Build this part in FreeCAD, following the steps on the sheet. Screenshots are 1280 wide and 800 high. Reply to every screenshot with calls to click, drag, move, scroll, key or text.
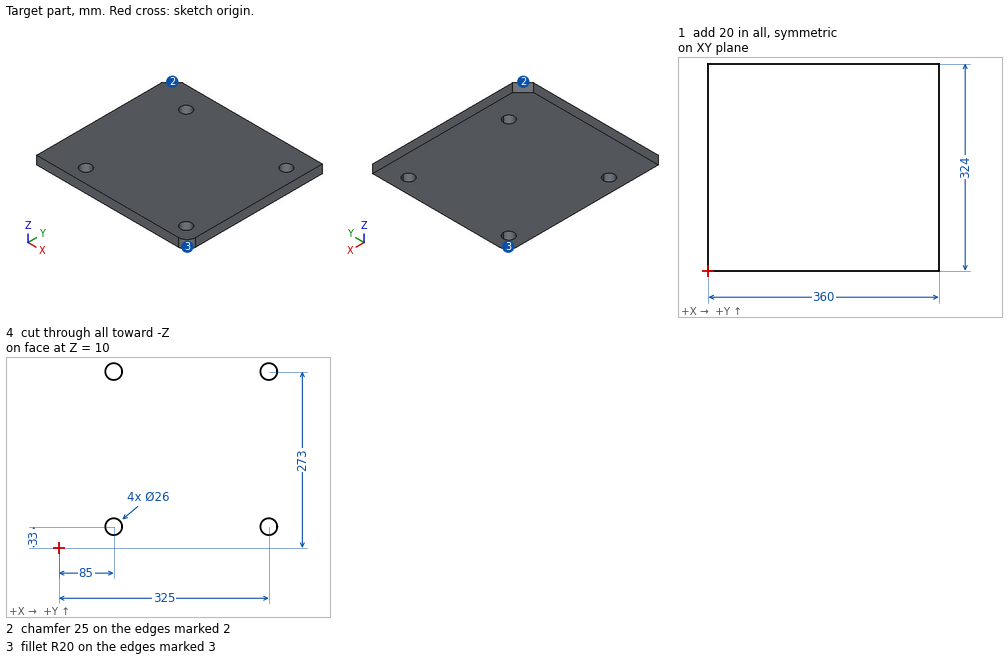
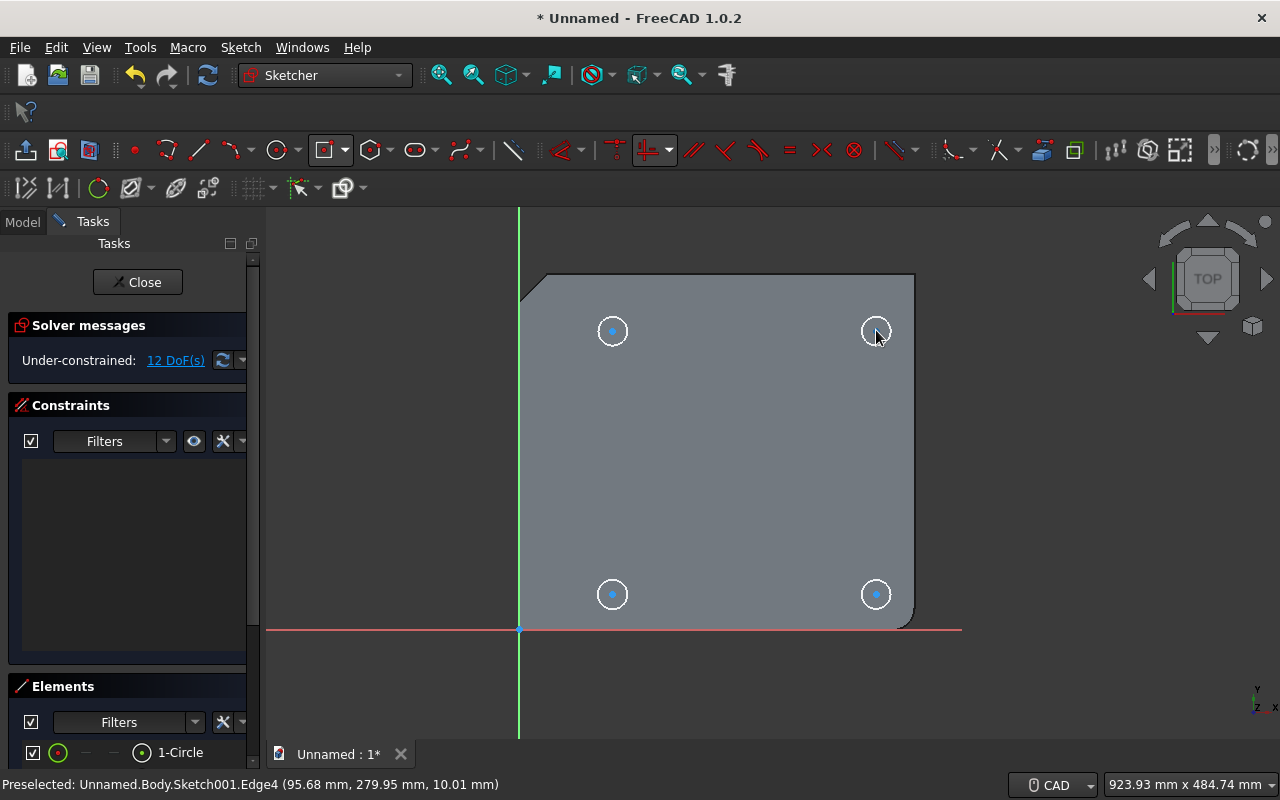
click(623, 584)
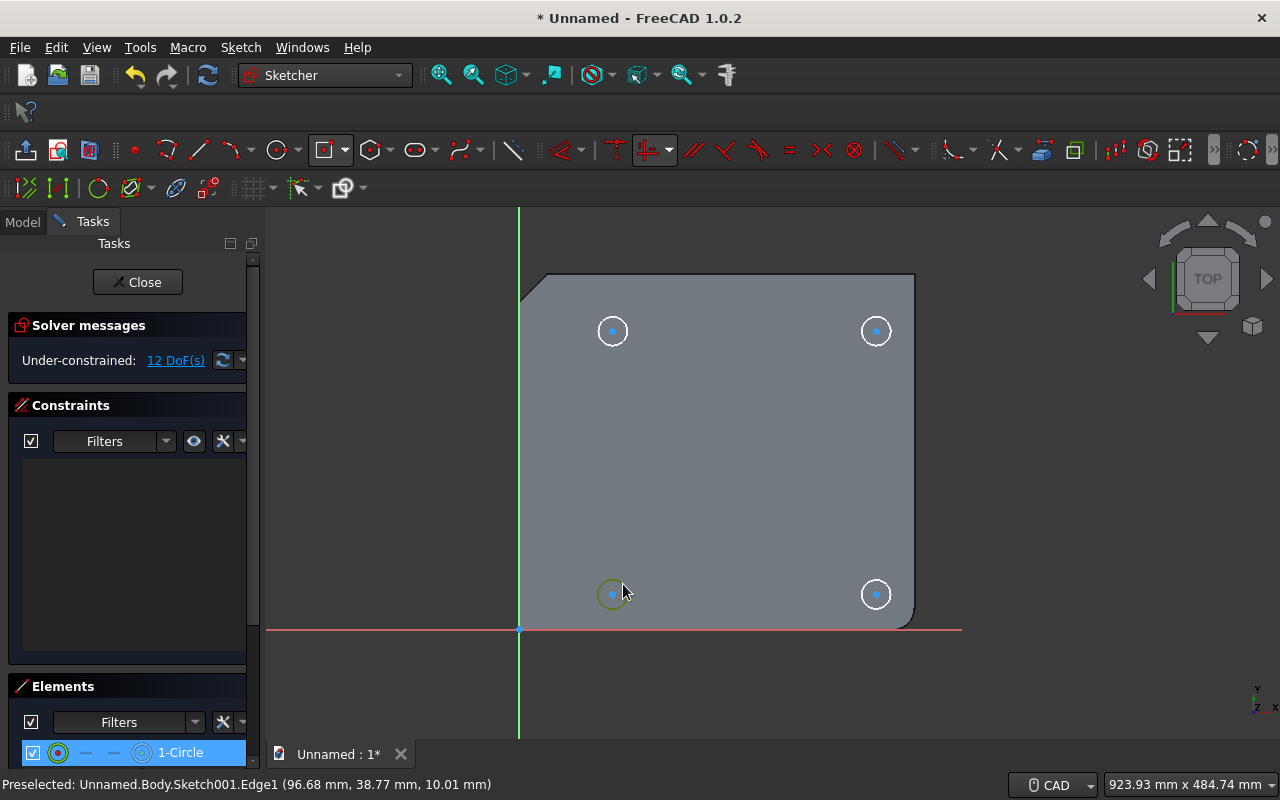
click(886, 584)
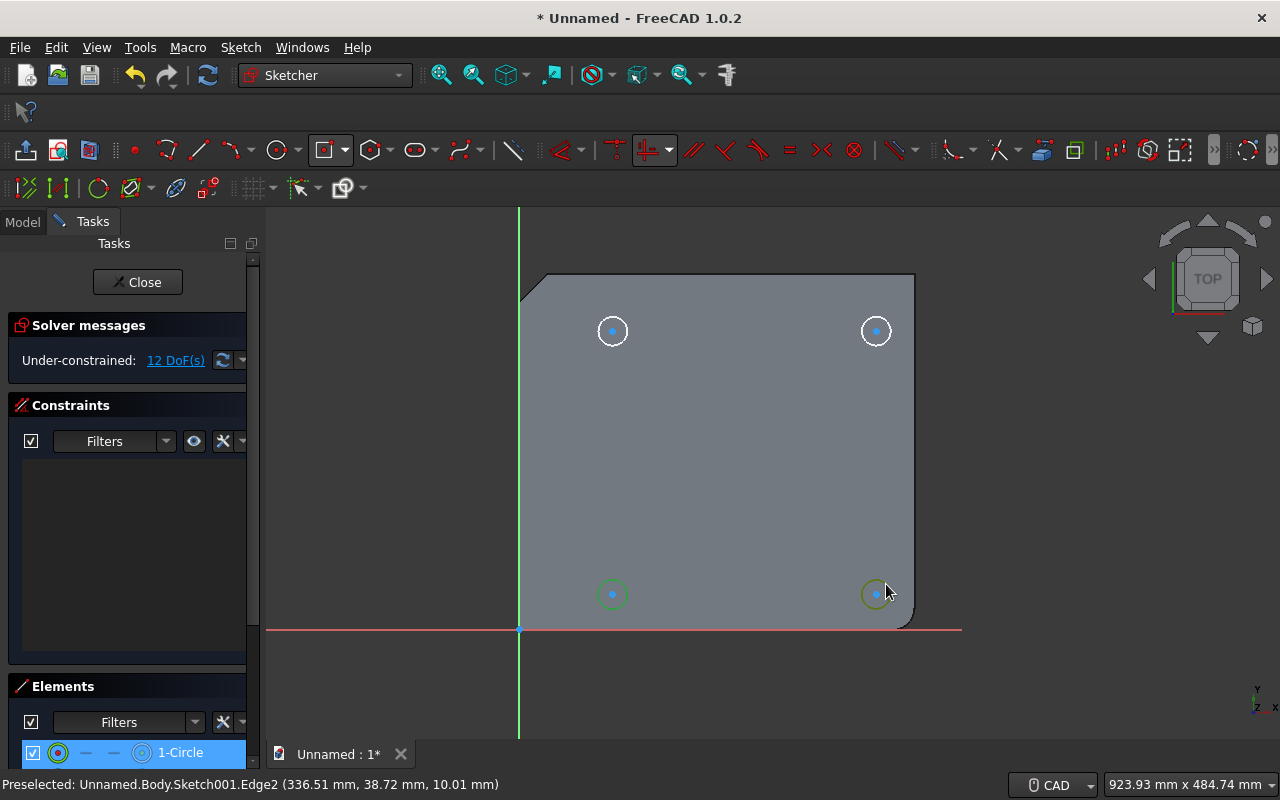
click(886, 321)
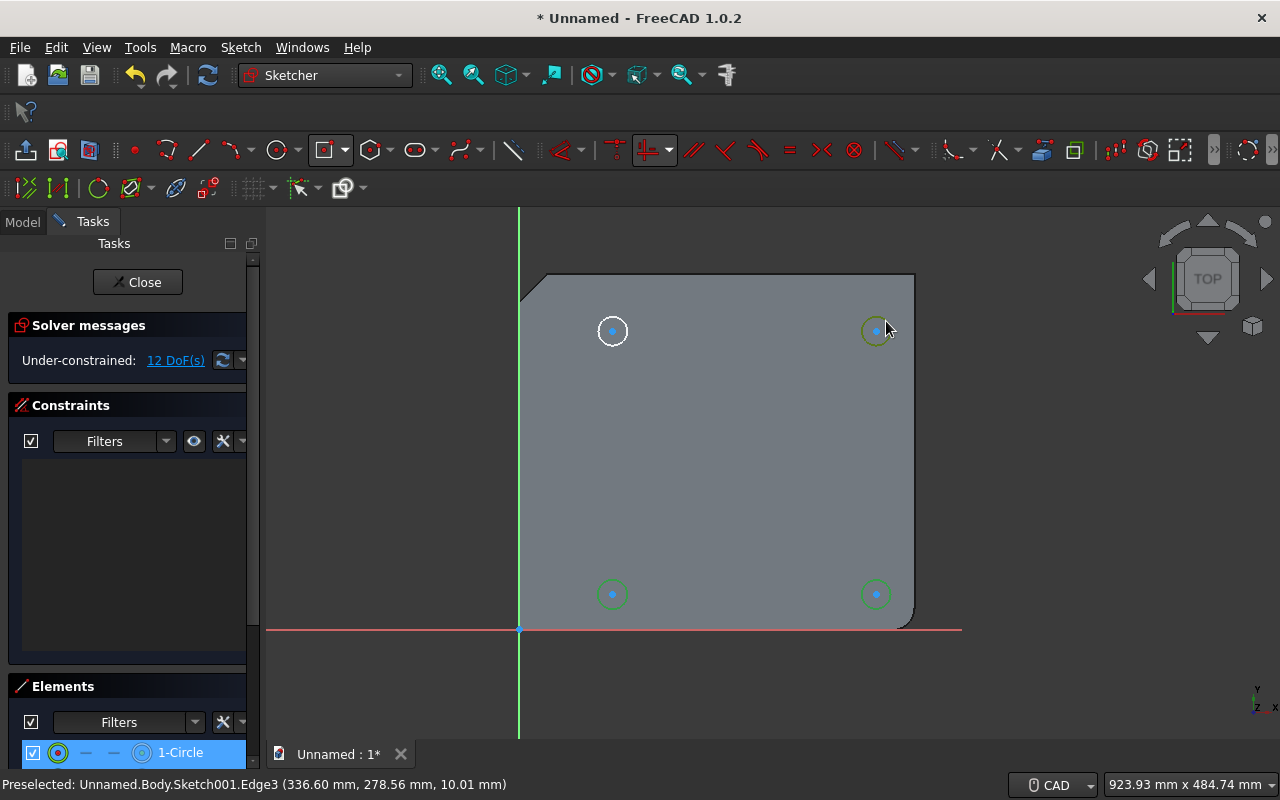
click(623, 321)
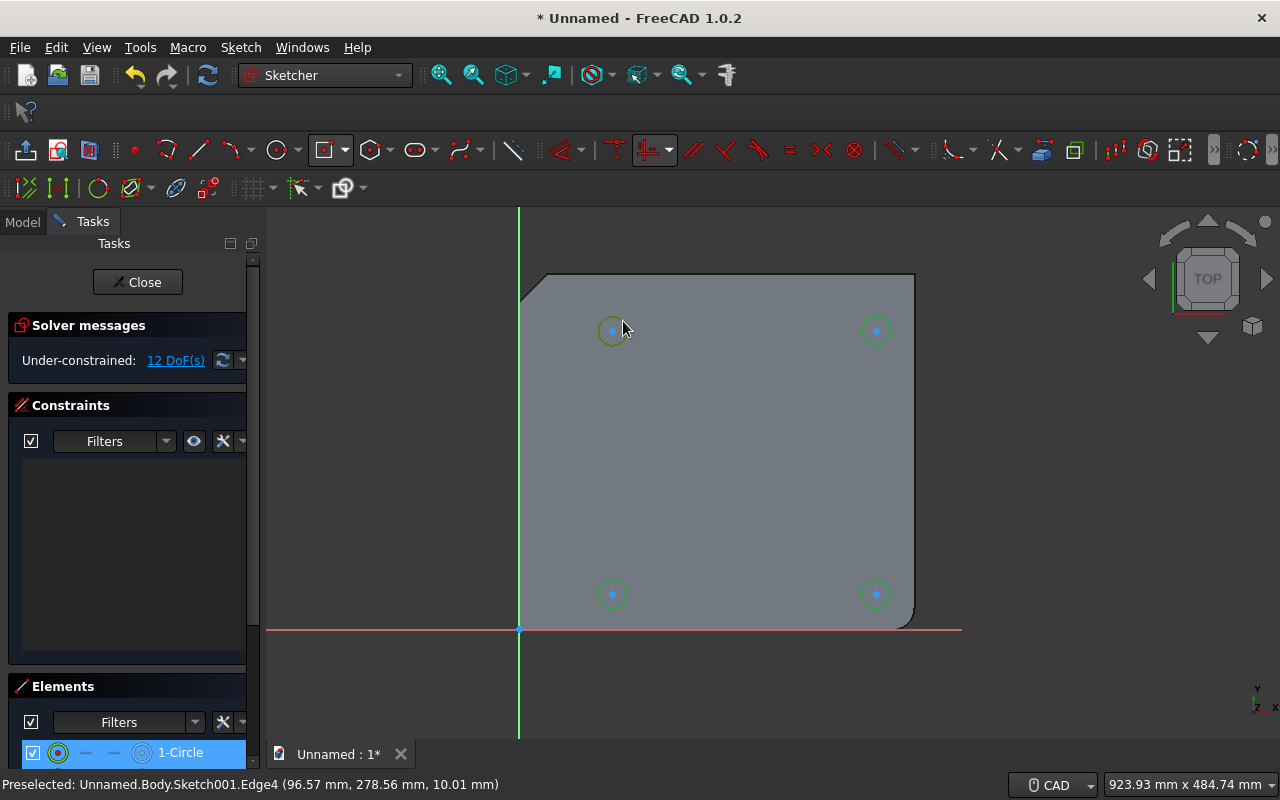
click(790, 150)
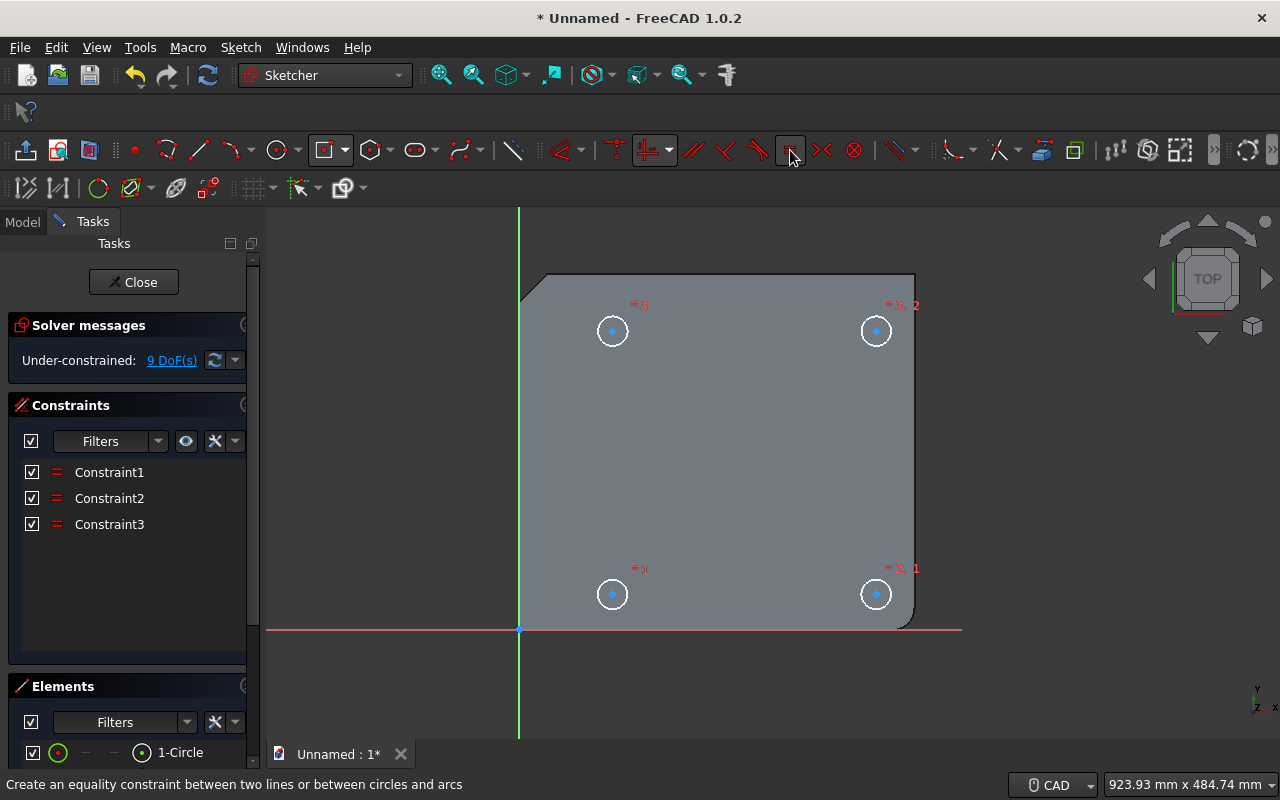
click(613, 595)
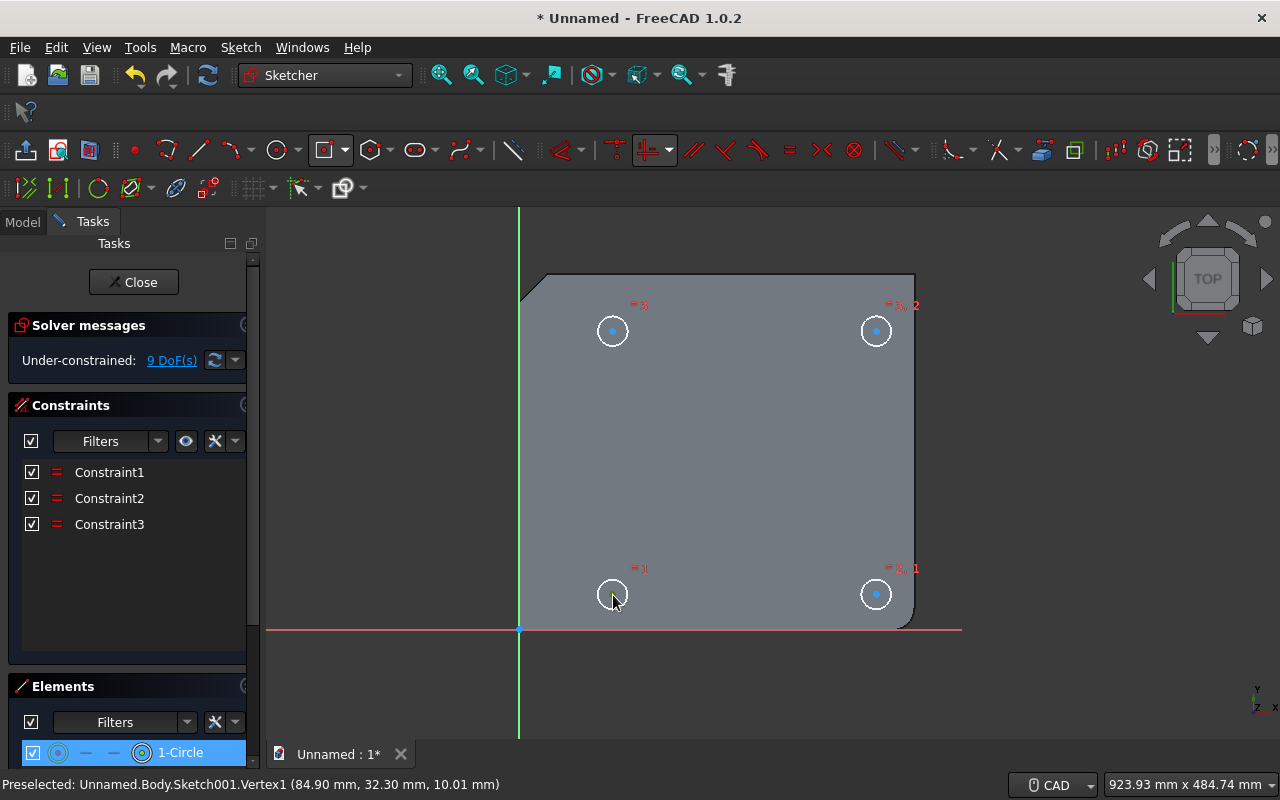
click(876, 594)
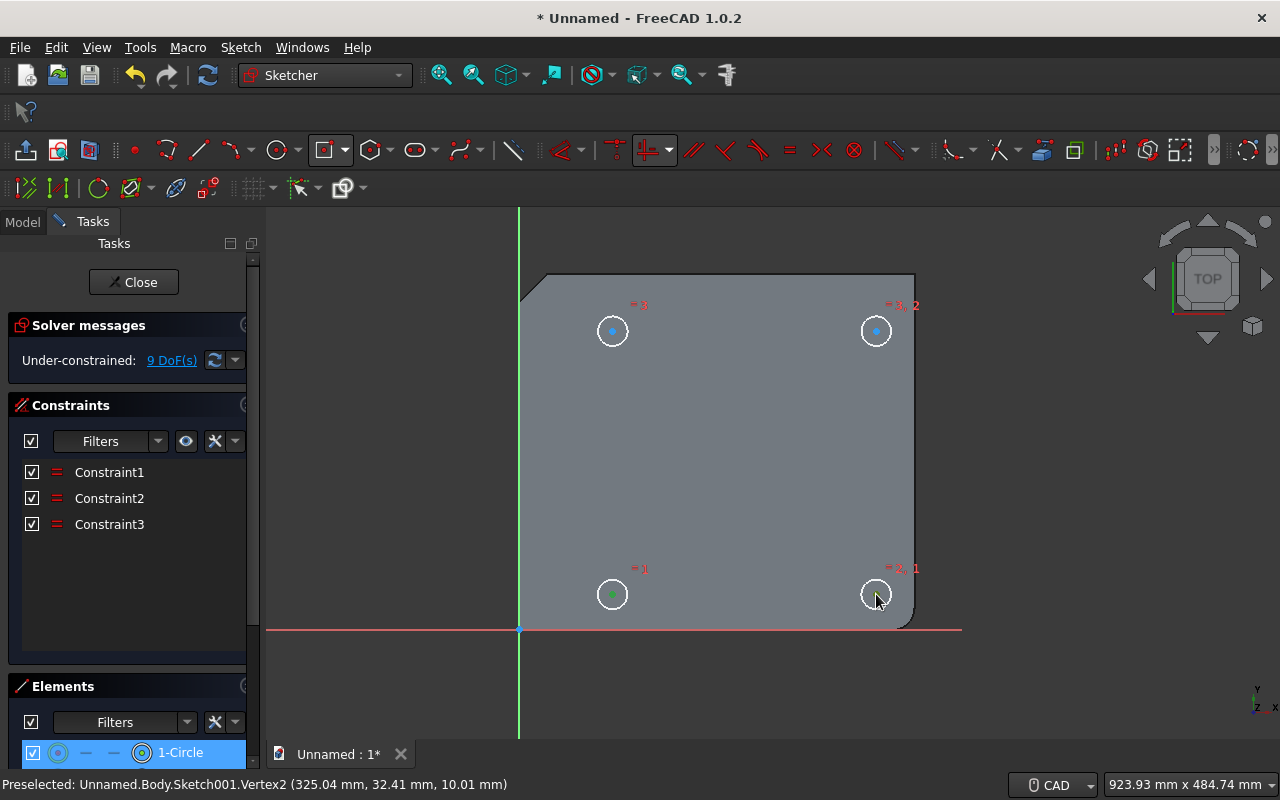
key(h)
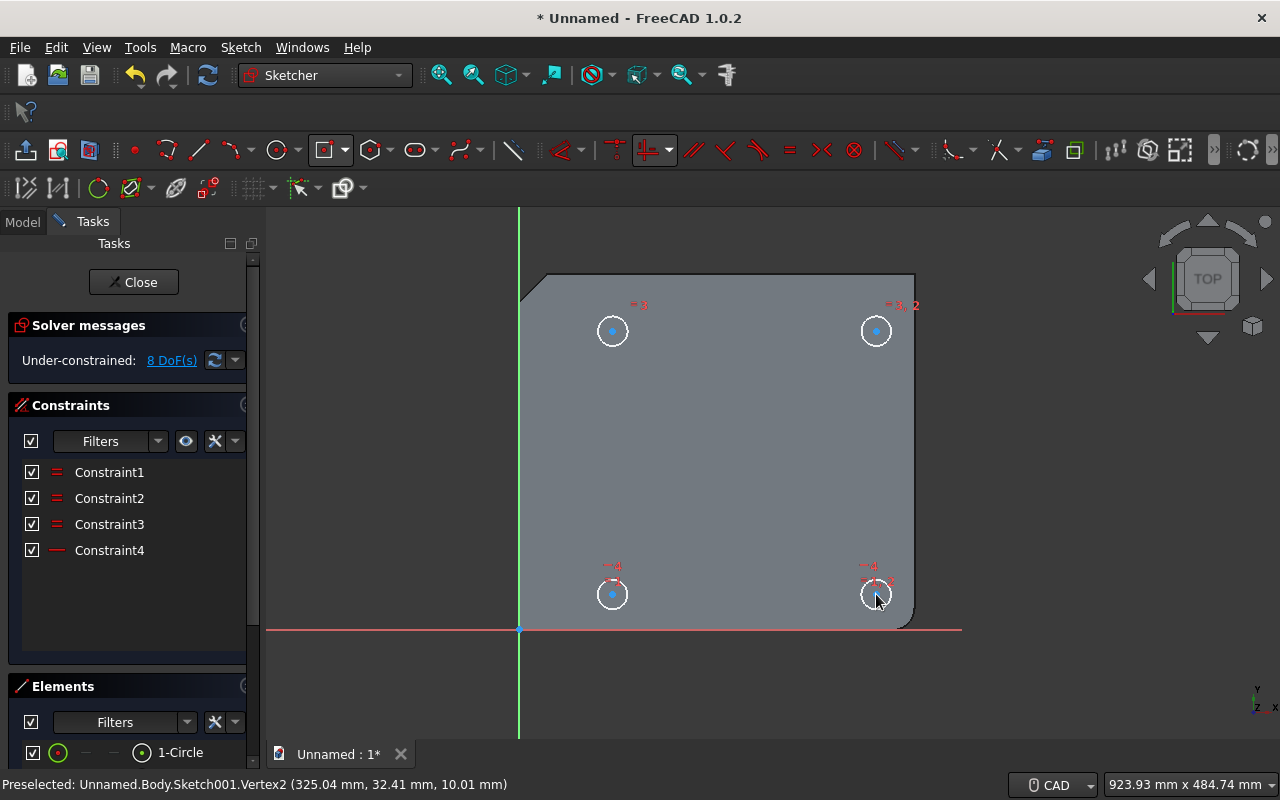
click(876, 595)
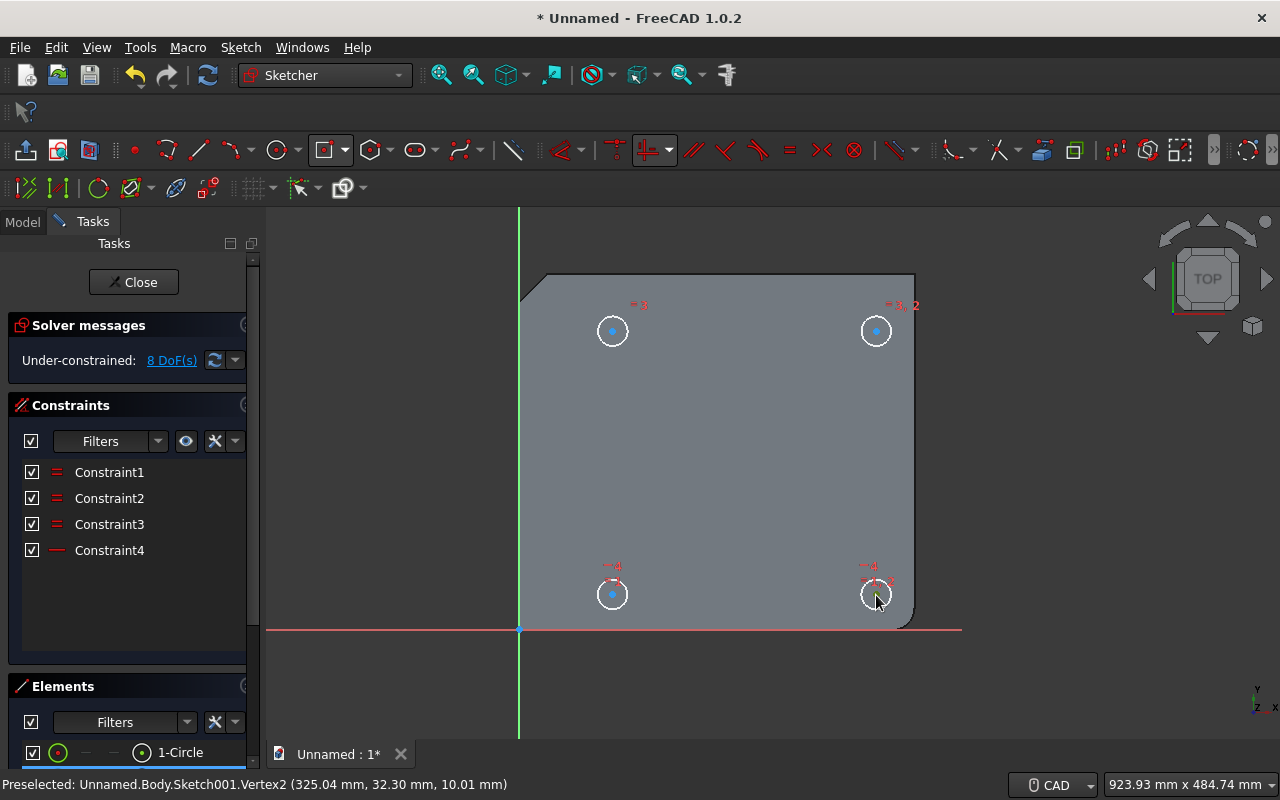
click(876, 331)